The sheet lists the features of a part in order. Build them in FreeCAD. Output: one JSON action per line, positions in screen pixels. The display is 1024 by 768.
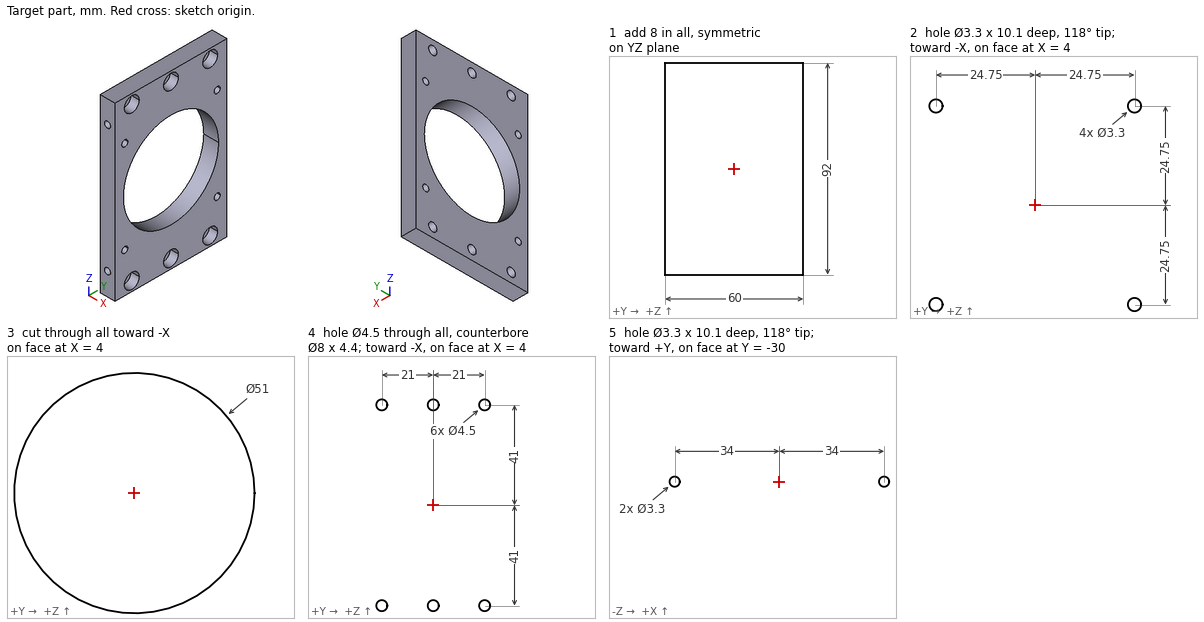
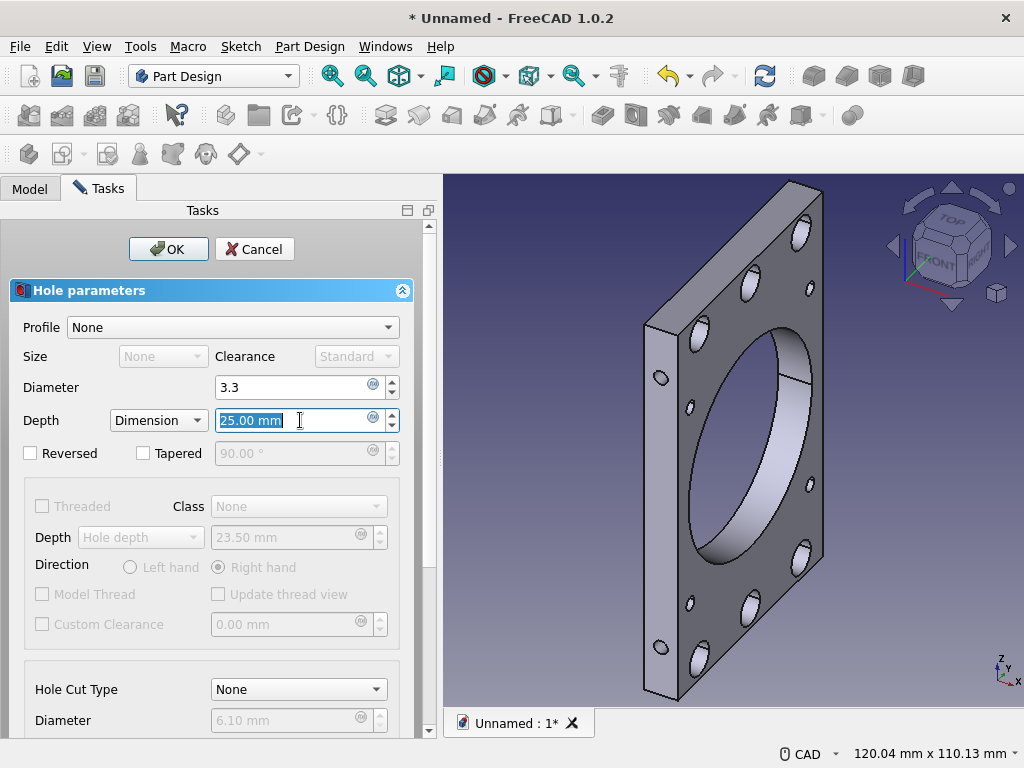
{"action": "type", "text": "10.1"}
{"action": "key", "text": "Tab"}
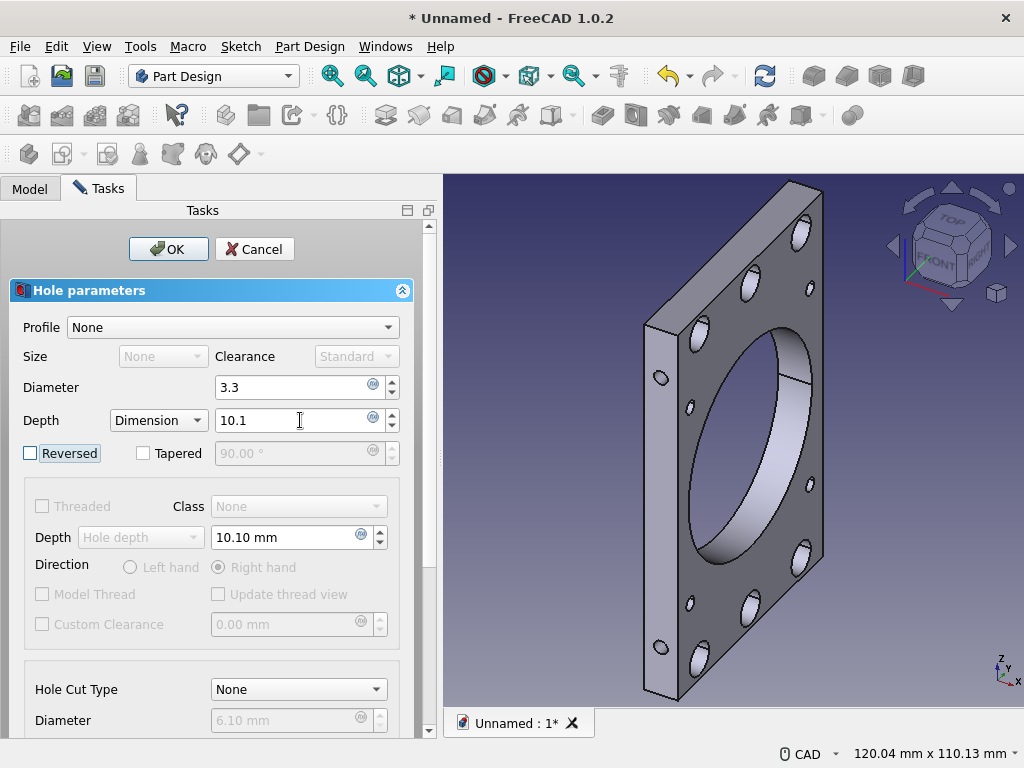
{"action": "left_click", "coordinate": [169, 249]}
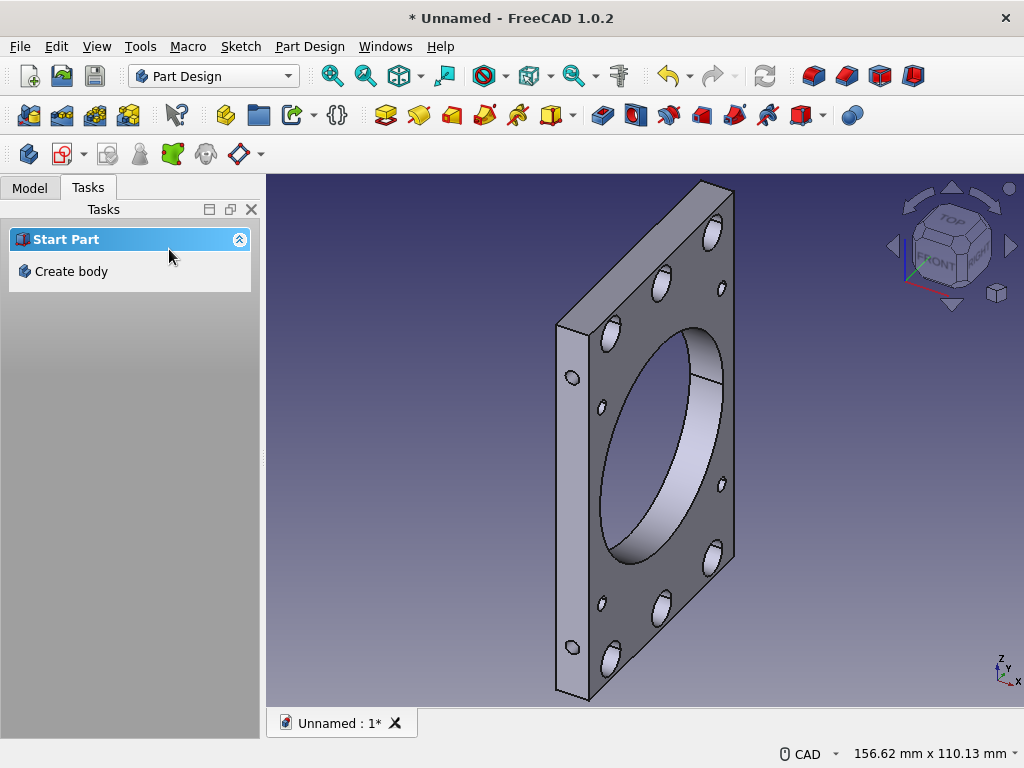
{"action": "key", "text": "0"}